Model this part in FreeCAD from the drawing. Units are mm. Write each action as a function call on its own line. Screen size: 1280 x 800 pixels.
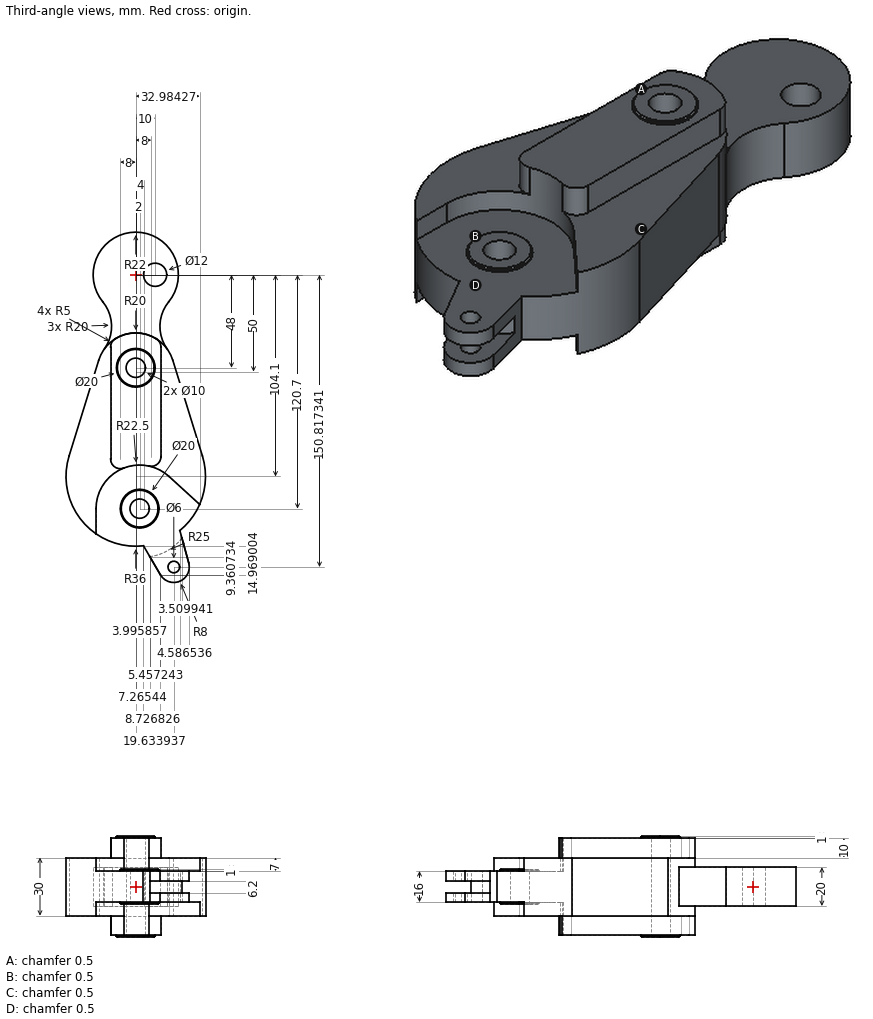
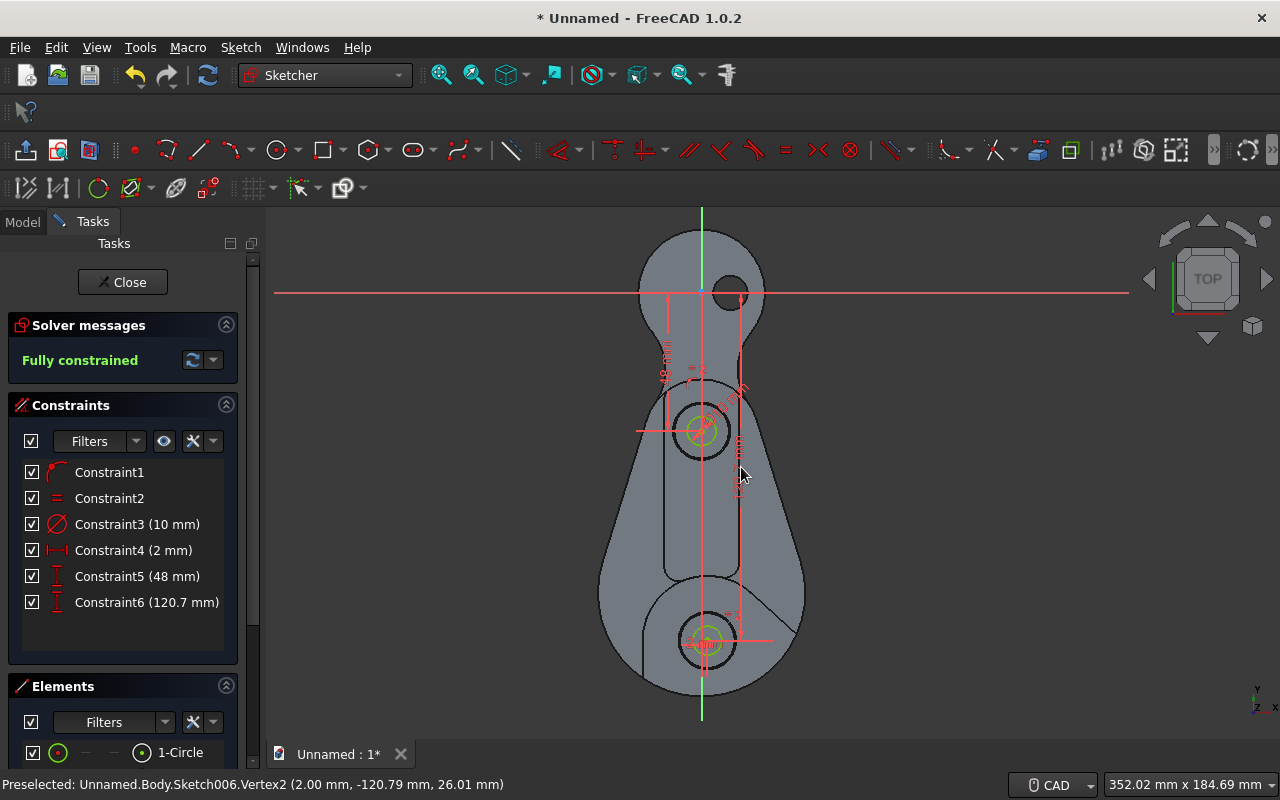
click(123, 282)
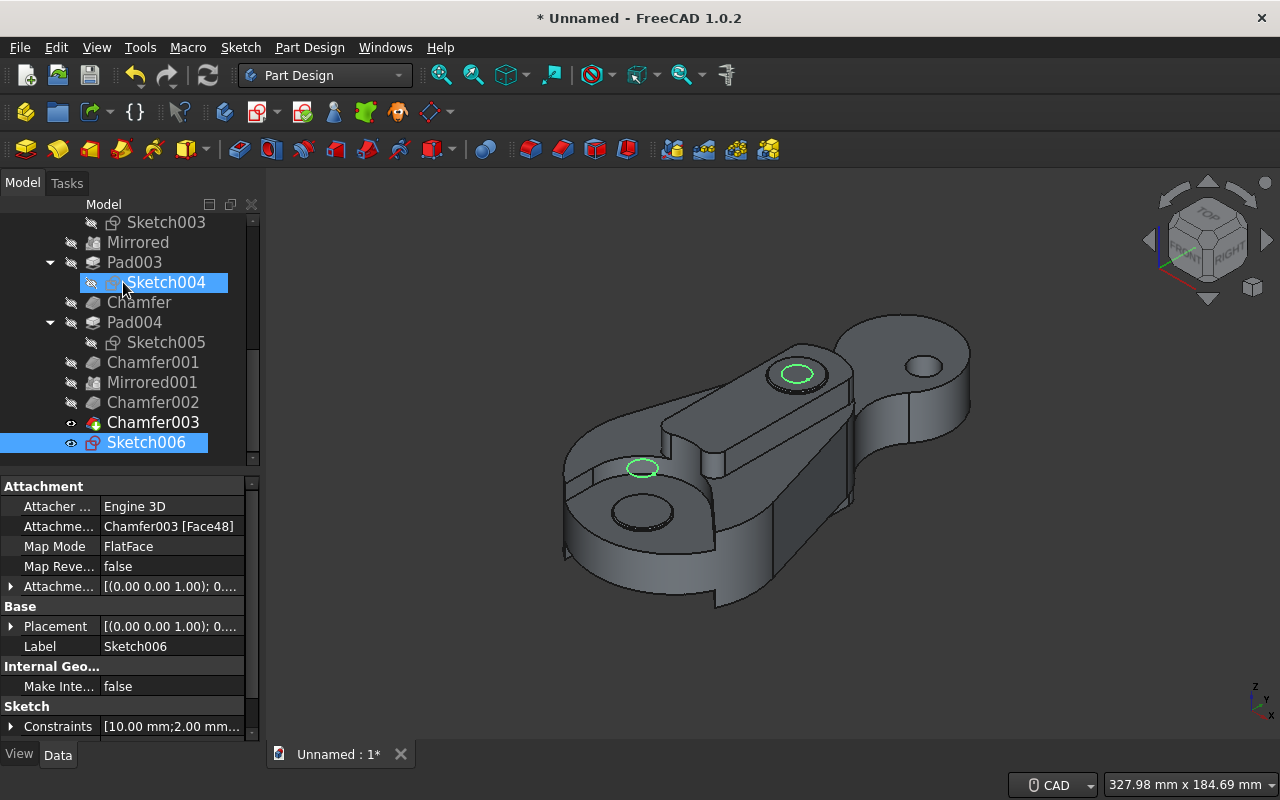
click(240, 150)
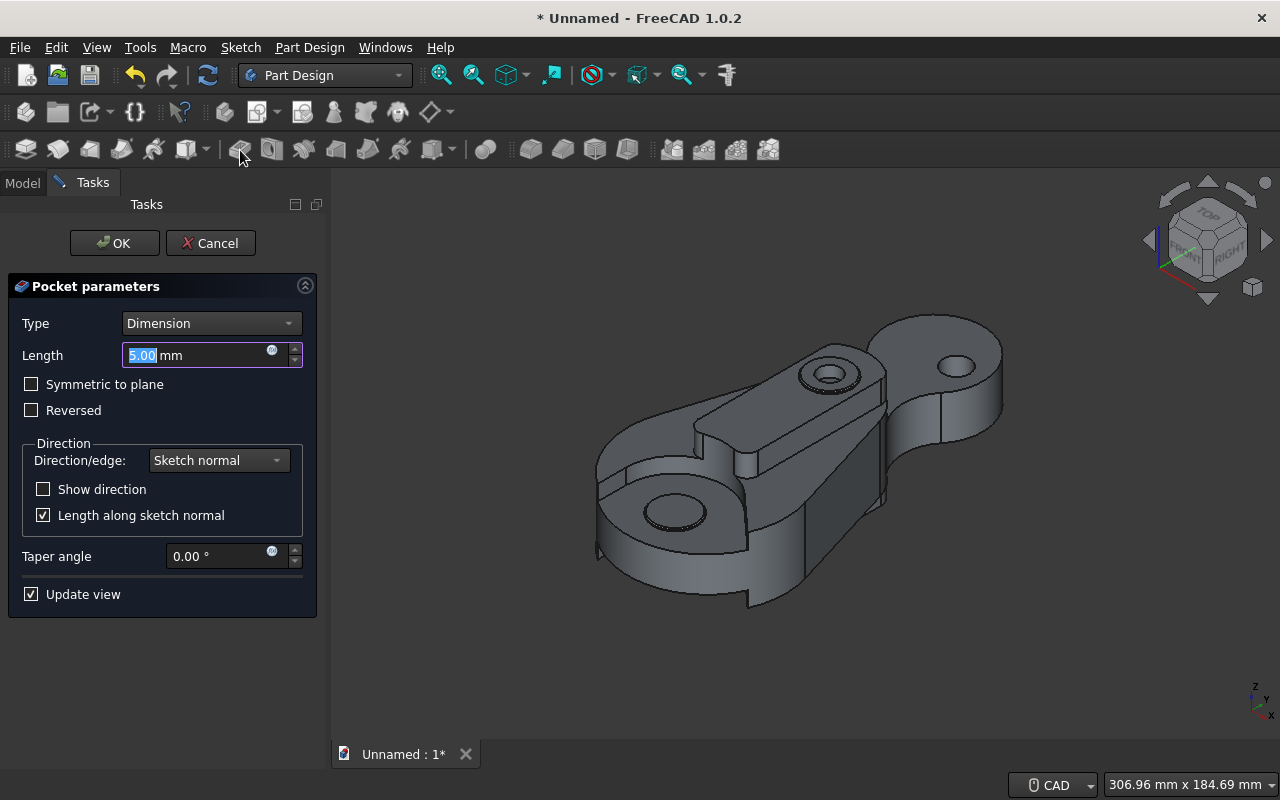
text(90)
key(Tab)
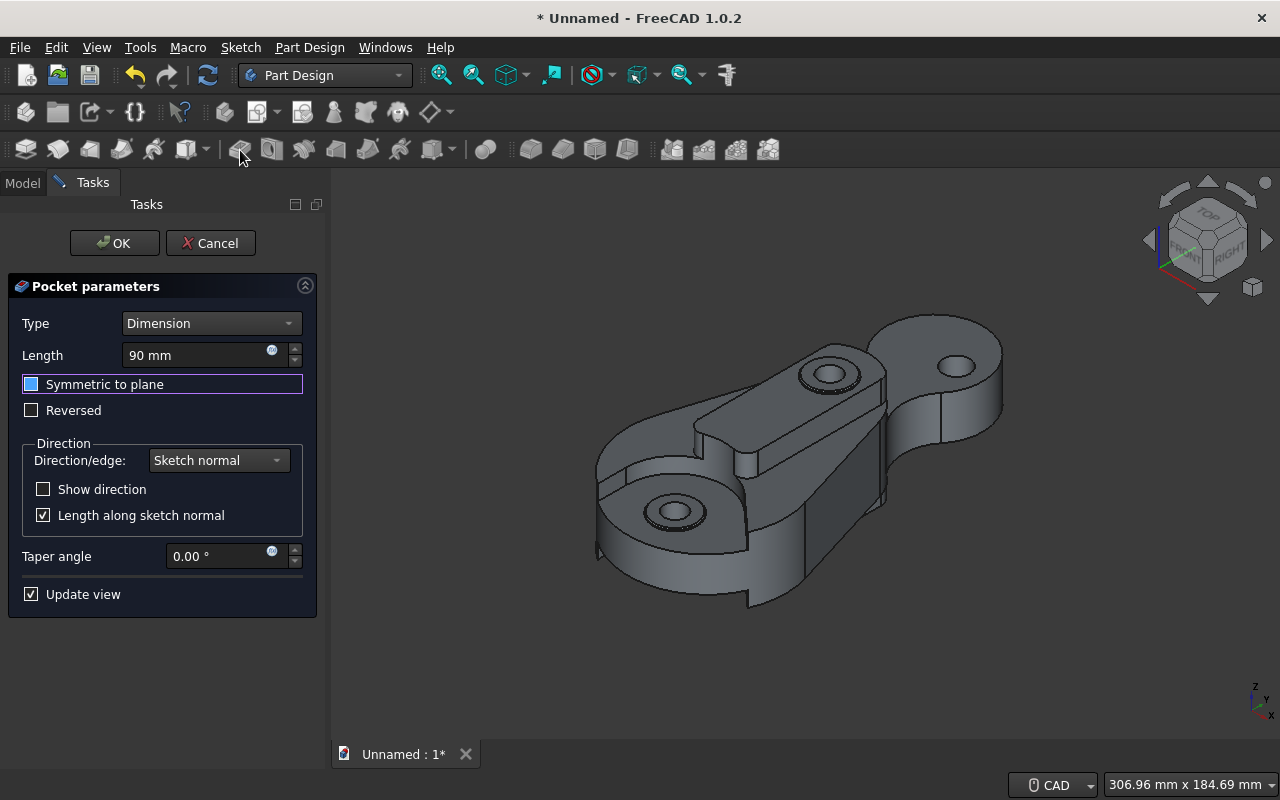
click(115, 243)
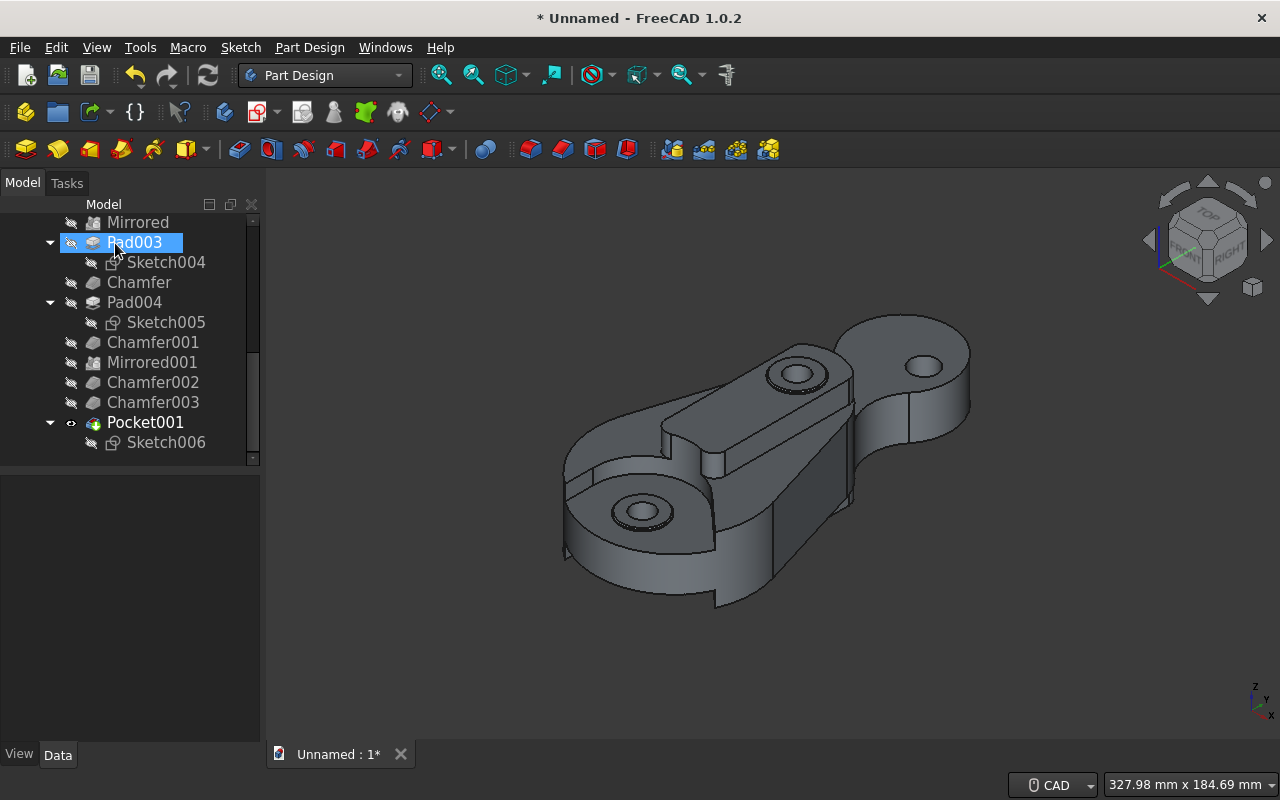
click(258, 112)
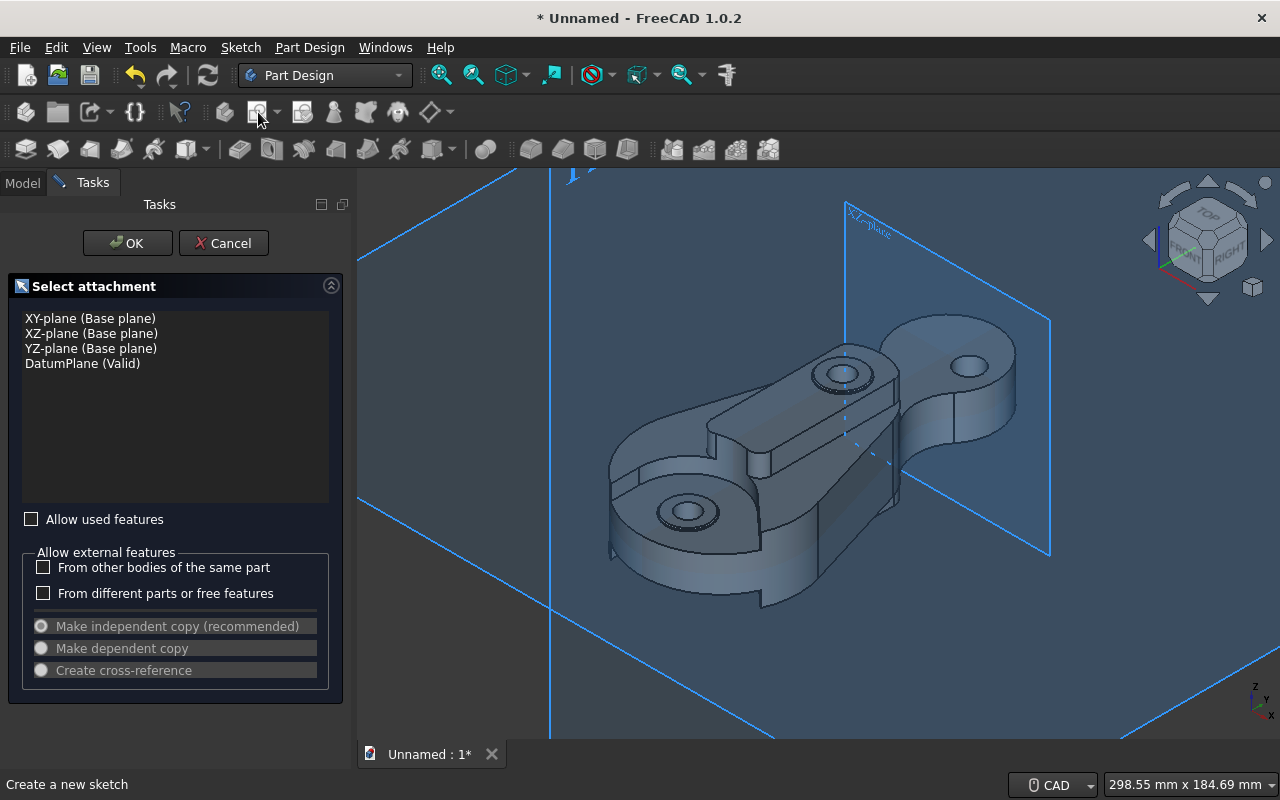
click(82, 318)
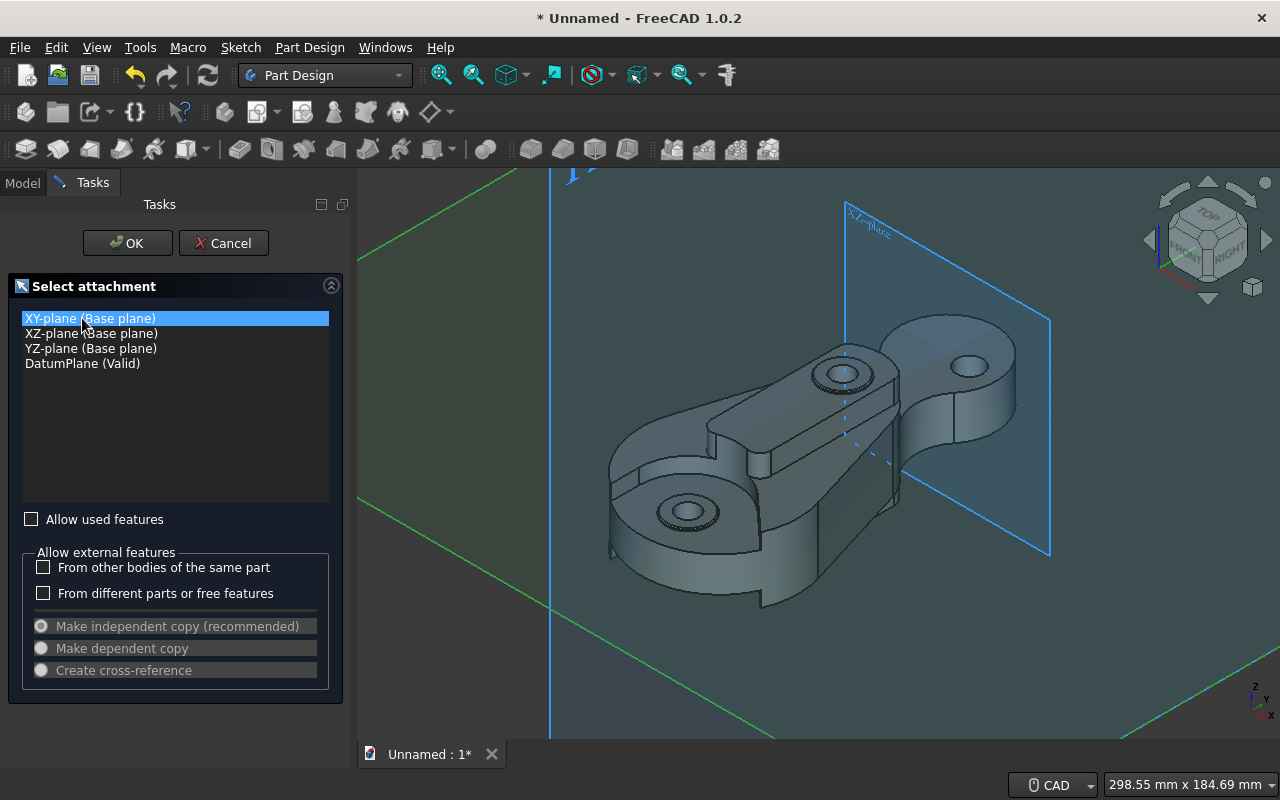
click(128, 243)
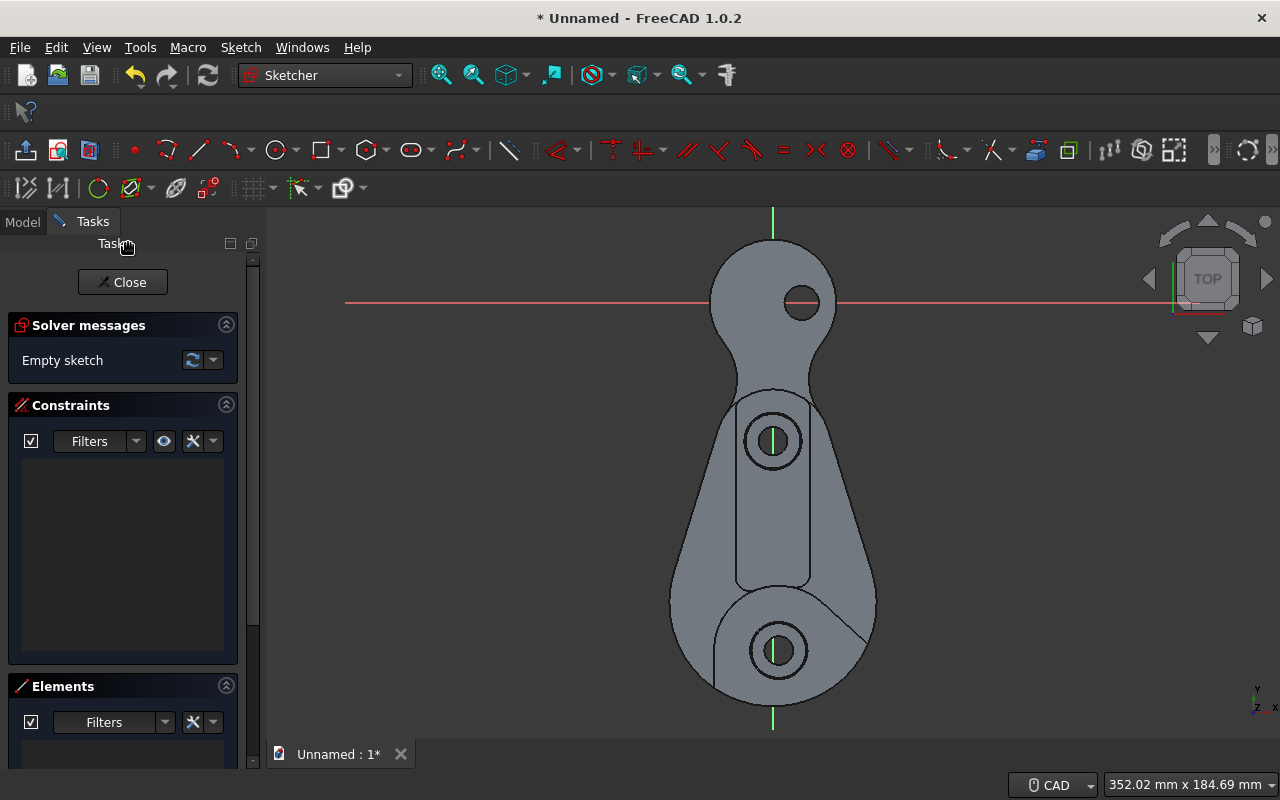
click(90, 150)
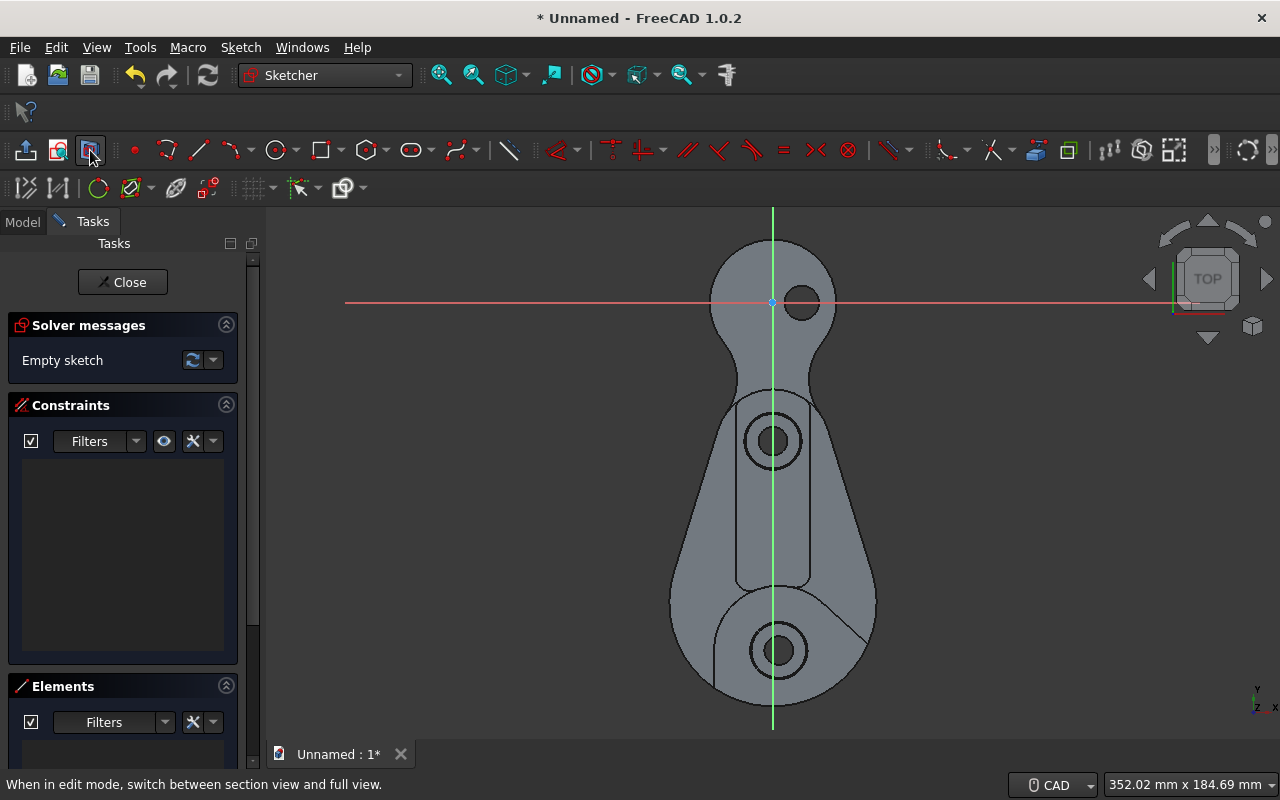
scroll(704, 473, down, 5)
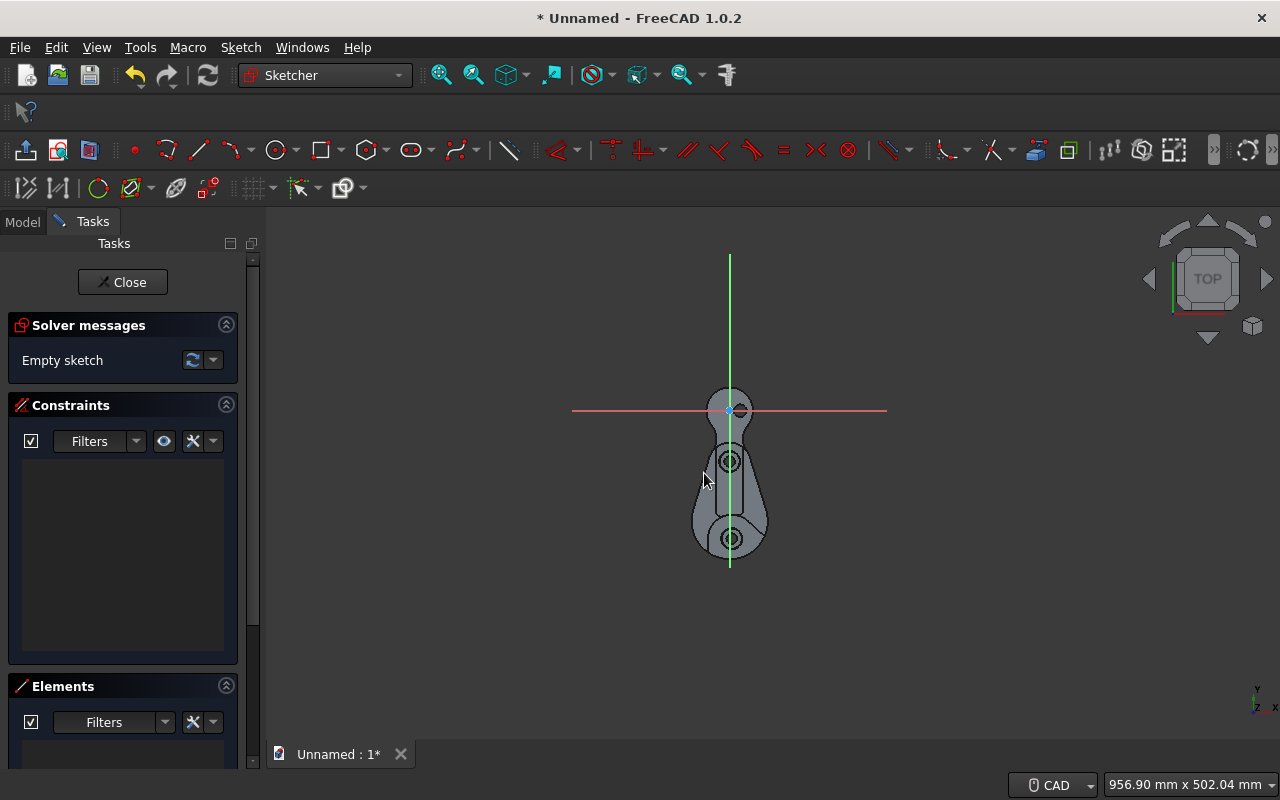
scroll(750, 574, up, 12)